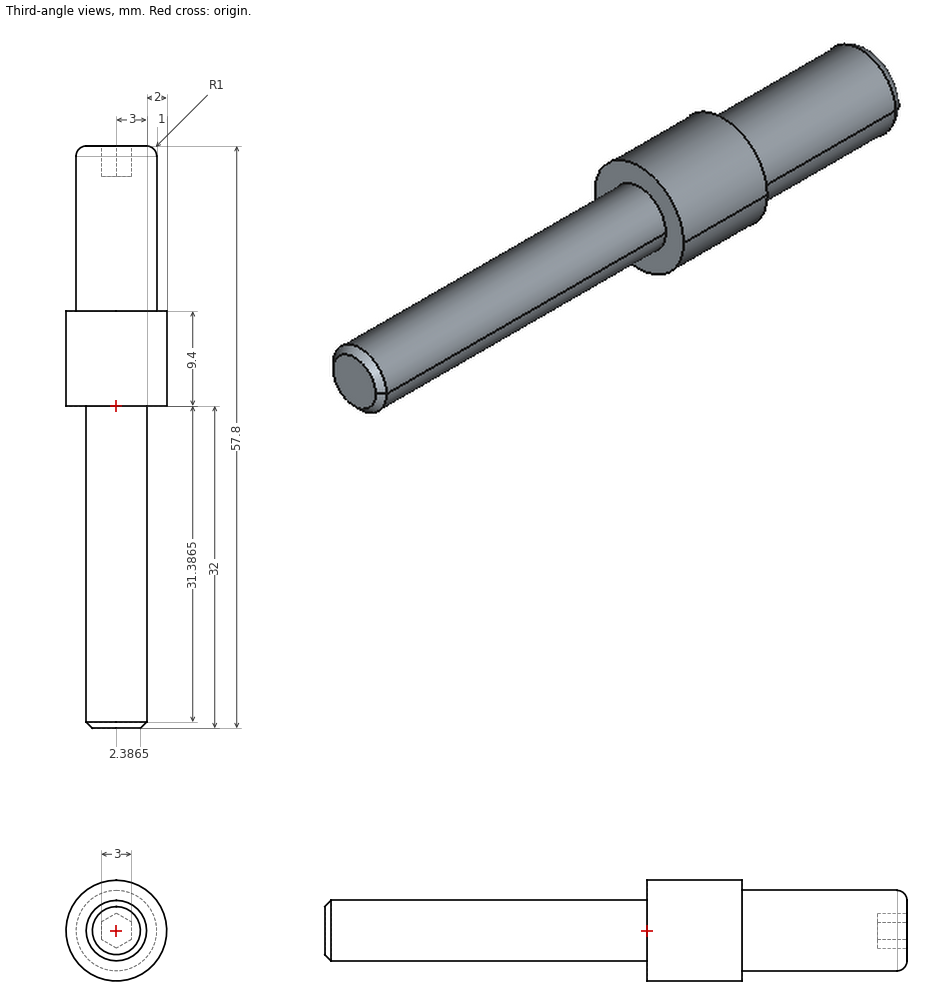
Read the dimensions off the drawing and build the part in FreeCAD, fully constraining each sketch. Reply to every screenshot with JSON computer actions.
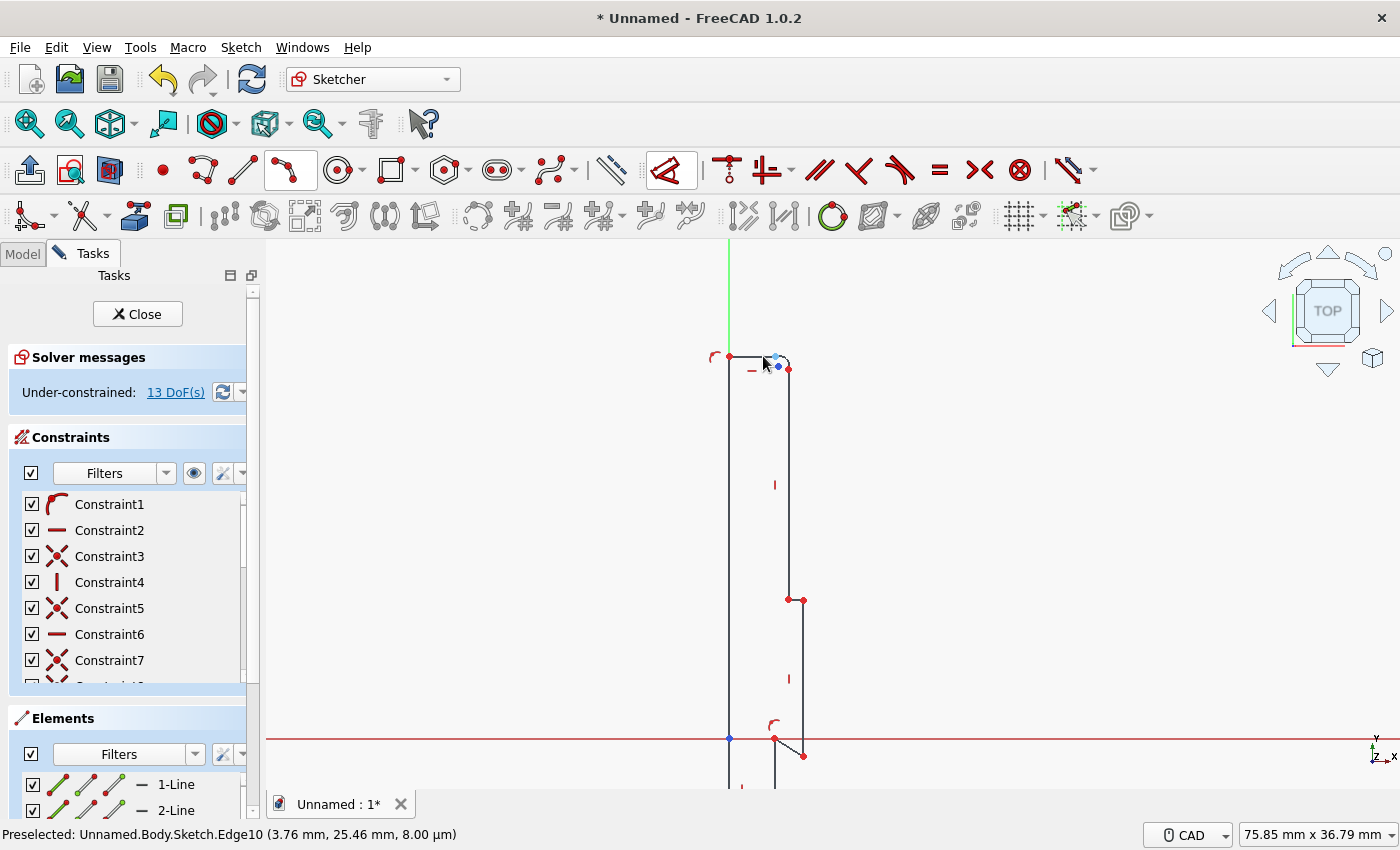
{"action": "left_click", "coordinate": [761, 357]}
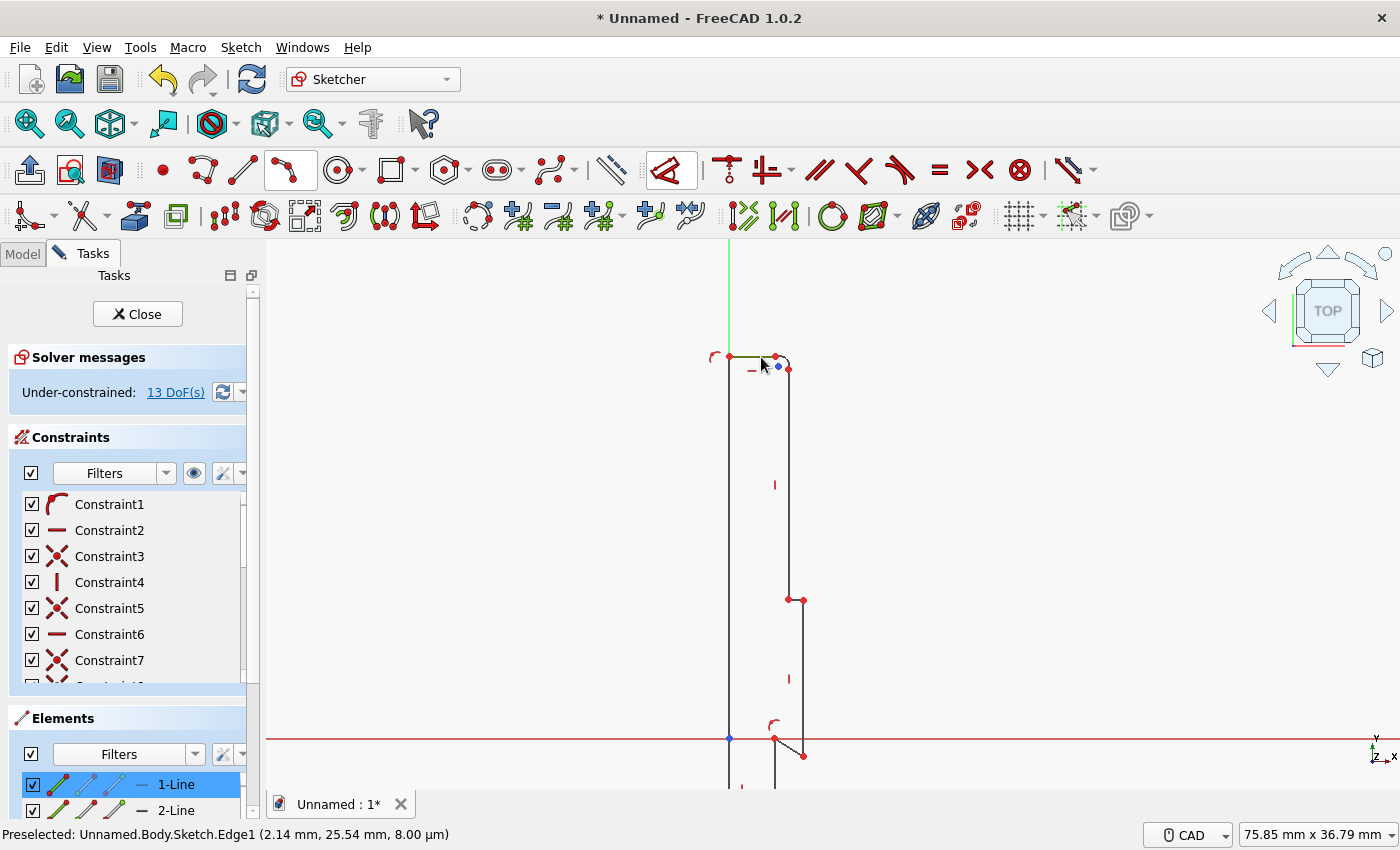
{"action": "scroll", "coordinate": [786, 359], "scroll_direction": "up", "scroll_amount": 2}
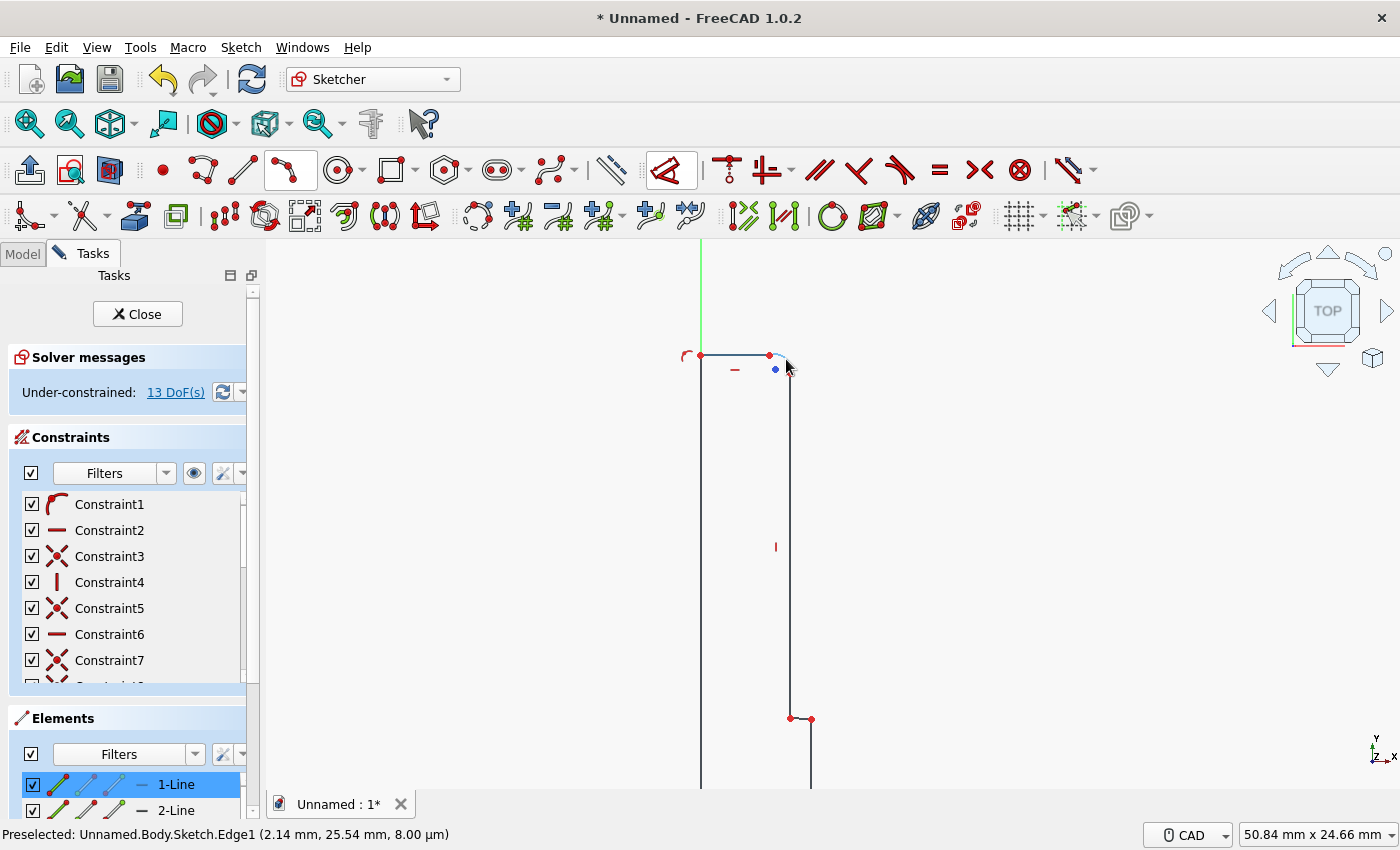
{"action": "left_click", "coordinate": [786, 358]}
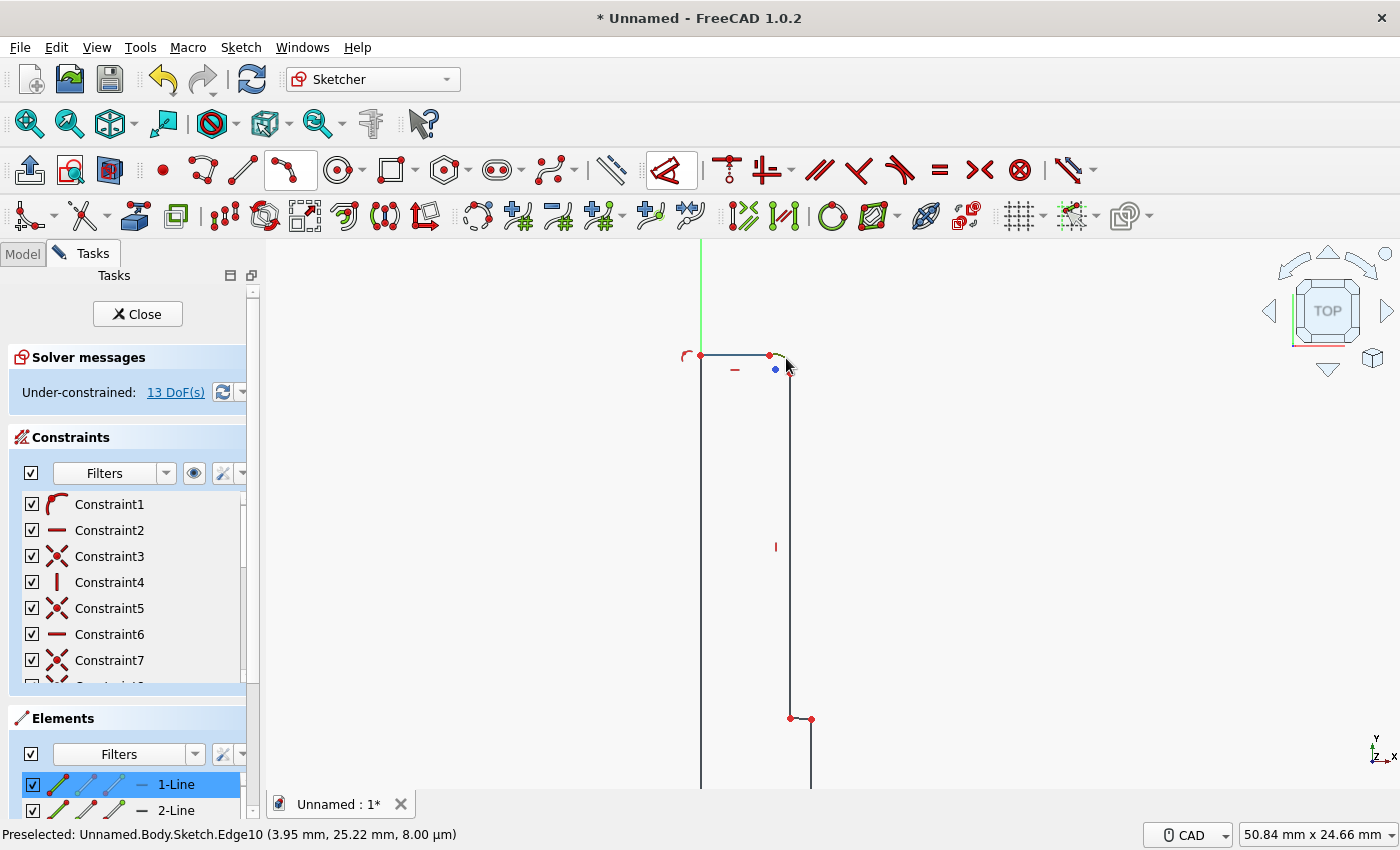
{"action": "left_click", "coordinate": [900, 170]}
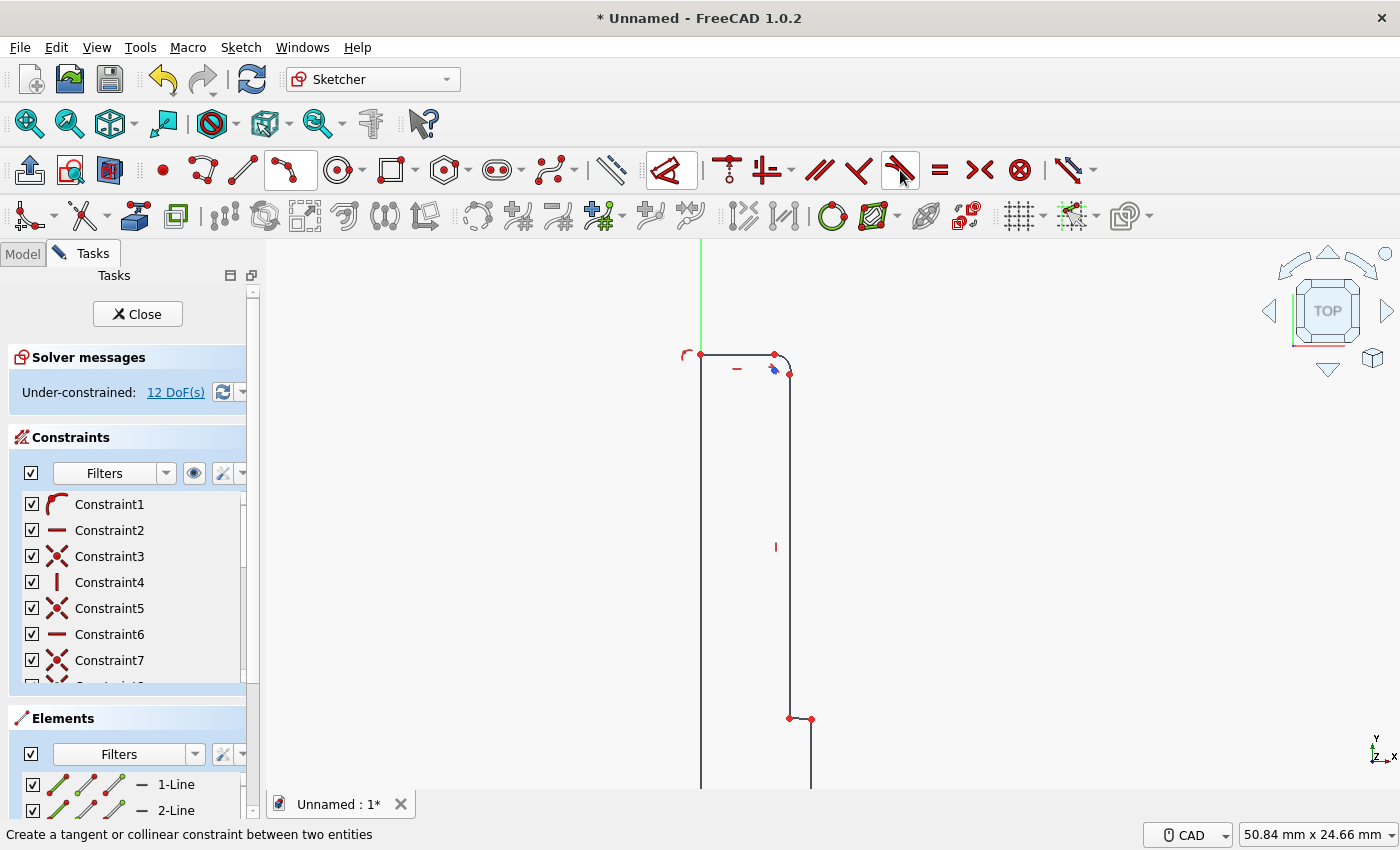
{"action": "scroll", "coordinate": [767, 357], "scroll_direction": "down", "scroll_amount": 7}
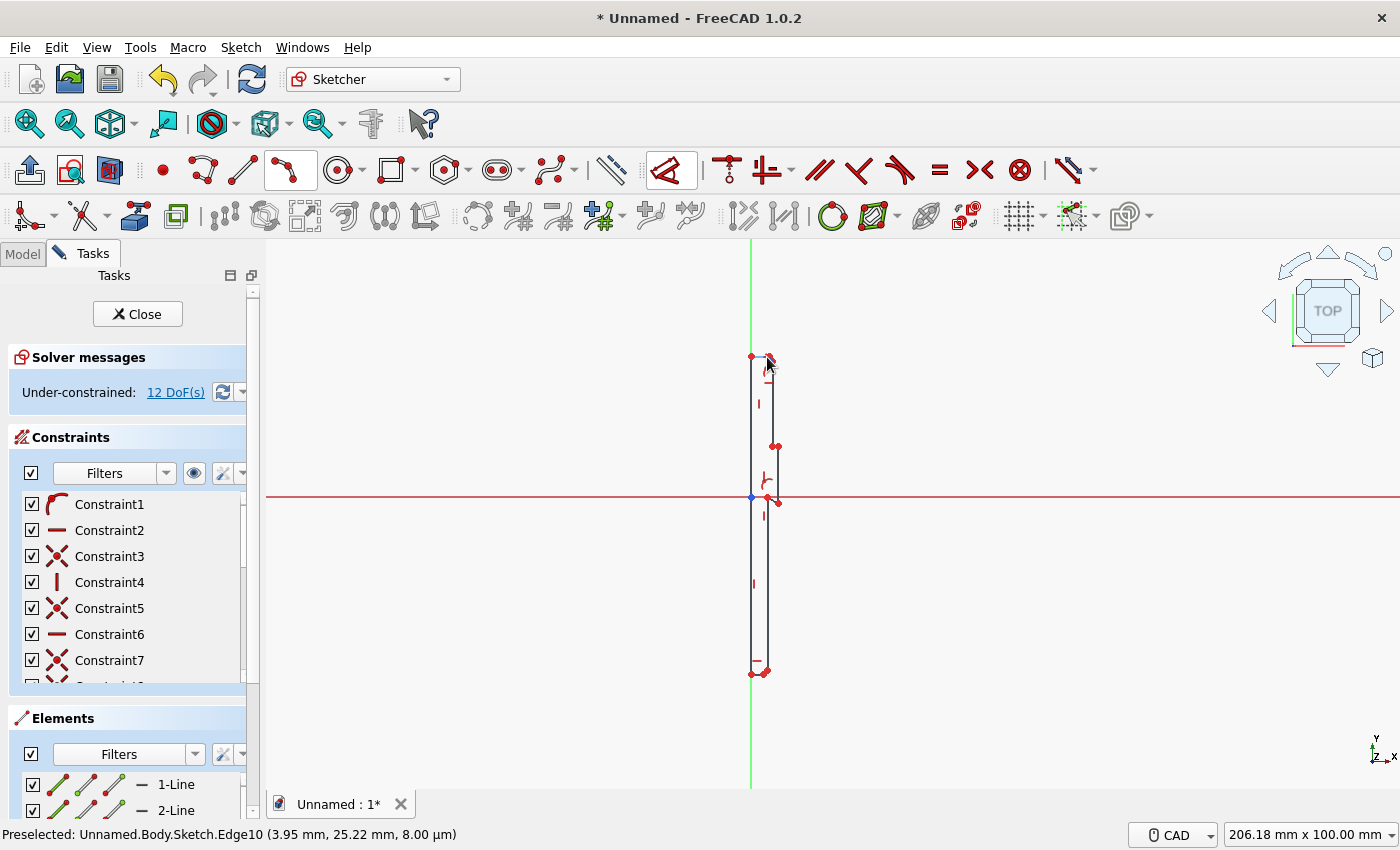
{"action": "left_click", "coordinate": [773, 421]}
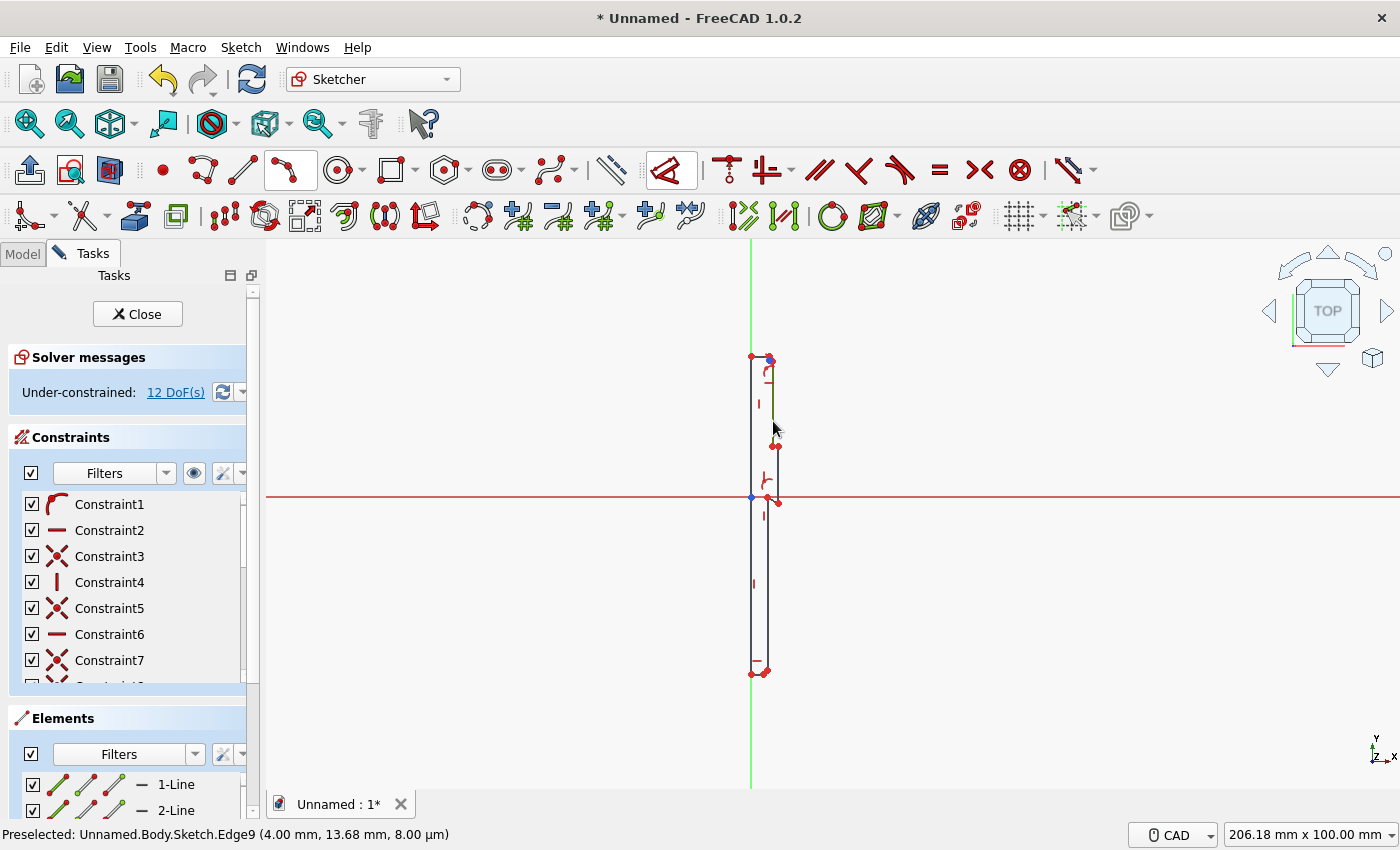
{"action": "scroll", "coordinate": [772, 358], "scroll_direction": "up", "scroll_amount": 7}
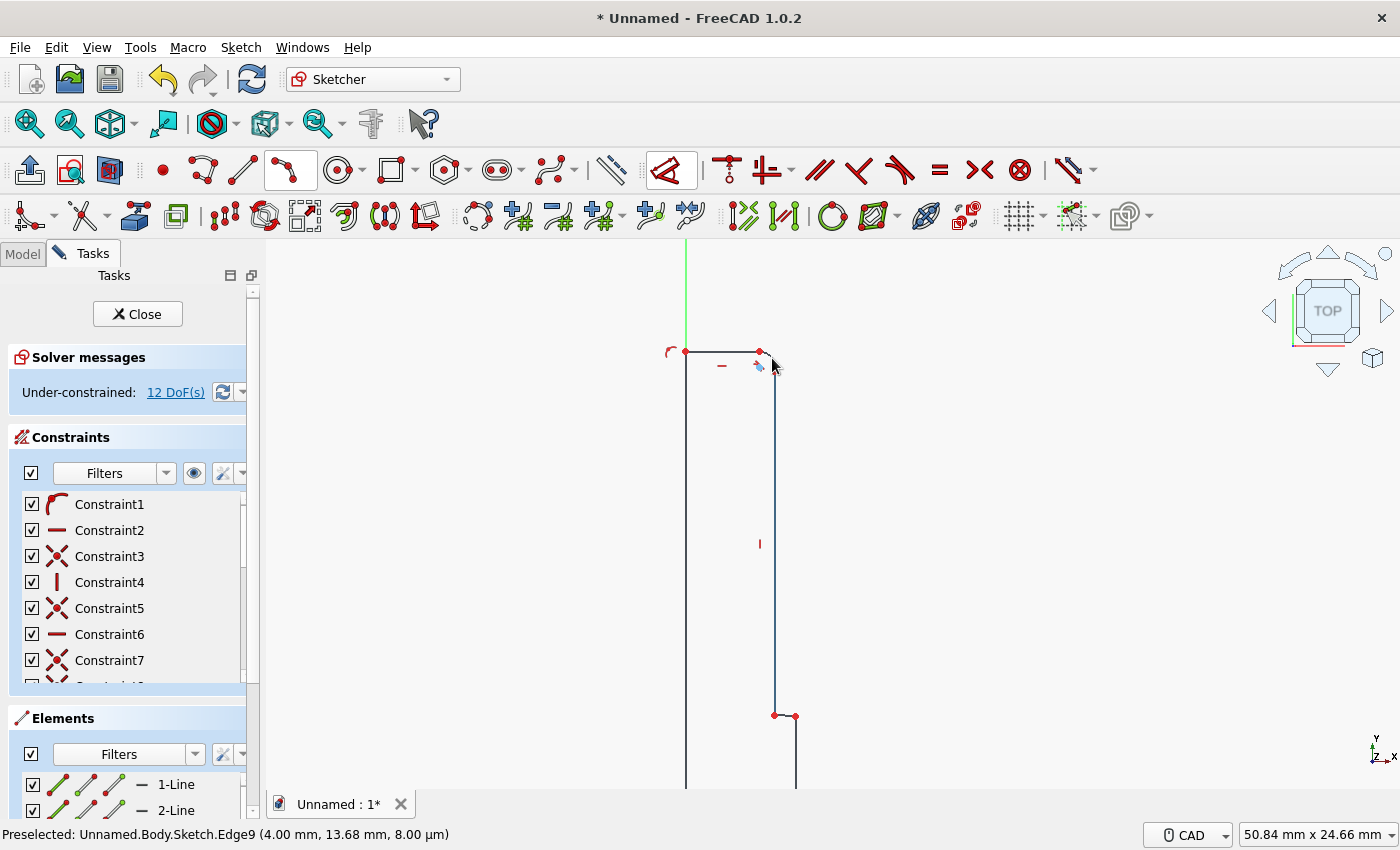
{"action": "left_click", "coordinate": [772, 358]}